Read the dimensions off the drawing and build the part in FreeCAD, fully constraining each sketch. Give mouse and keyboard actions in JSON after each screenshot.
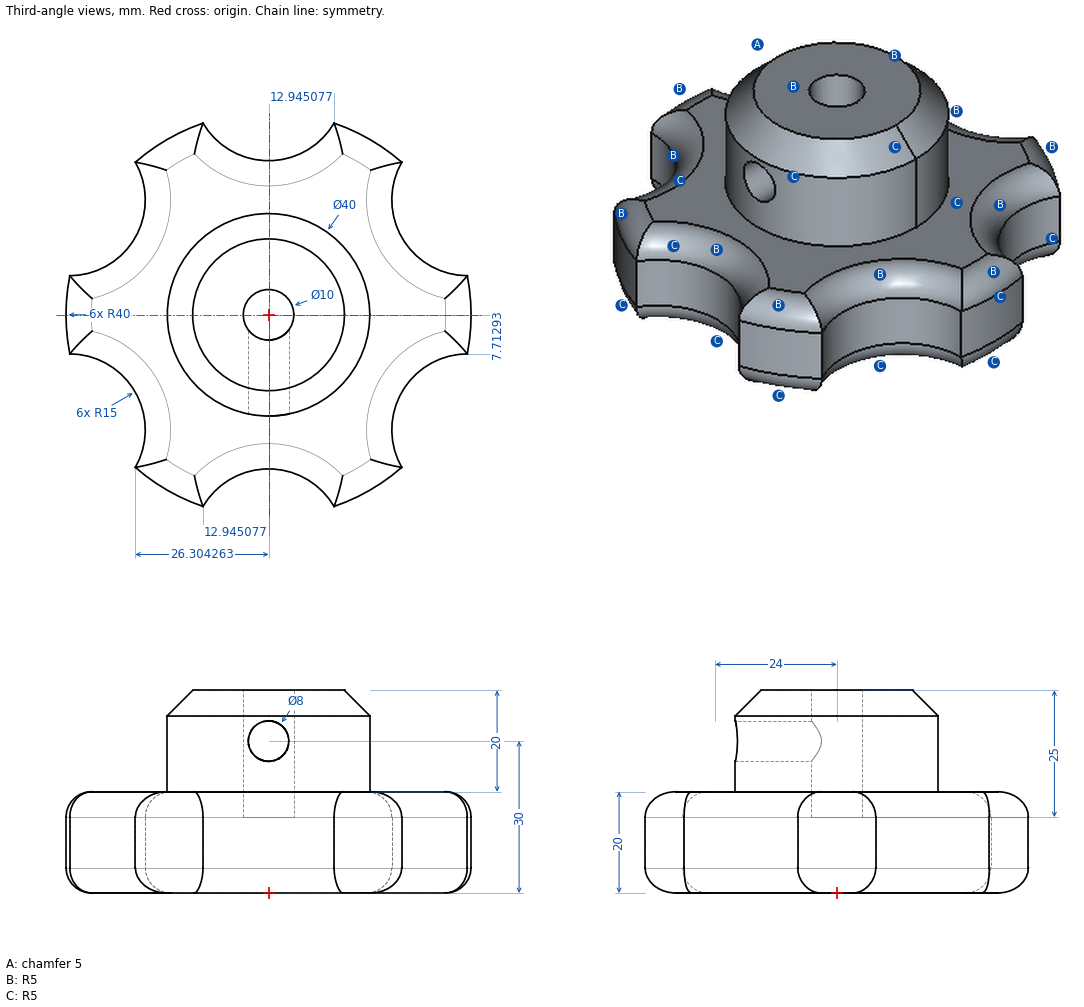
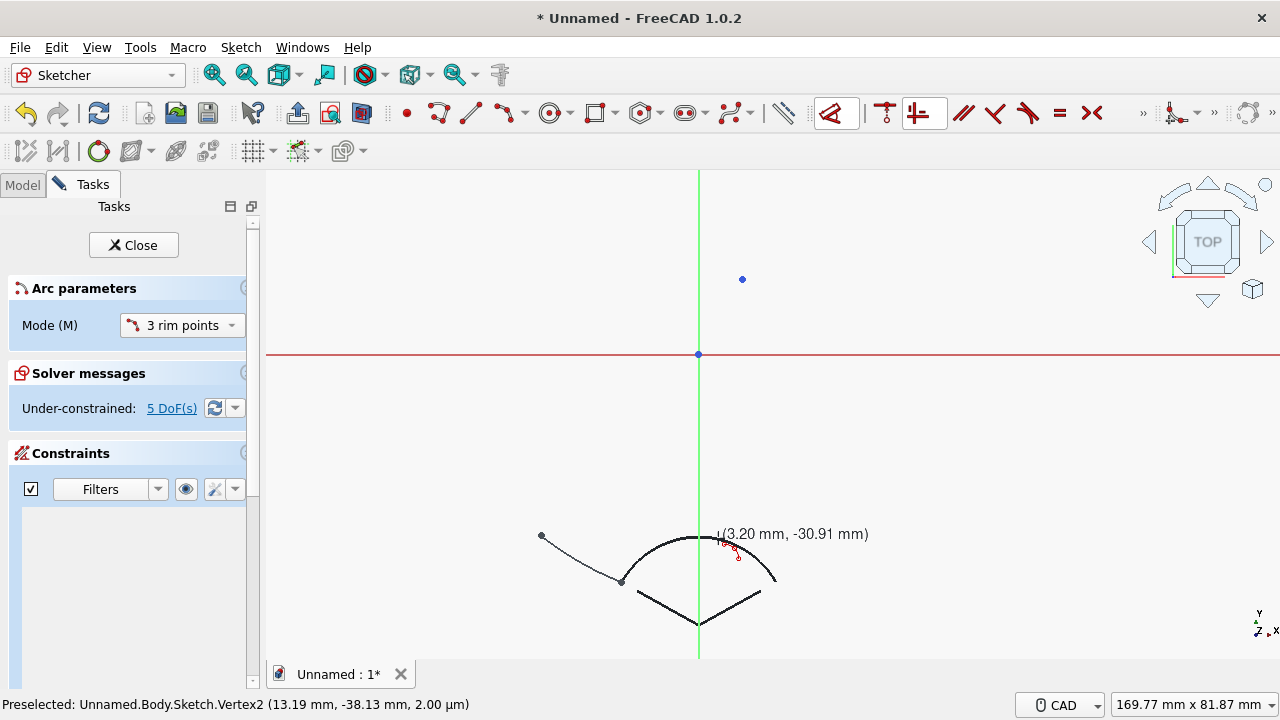
{"action": "left_click", "coordinate": [717, 538]}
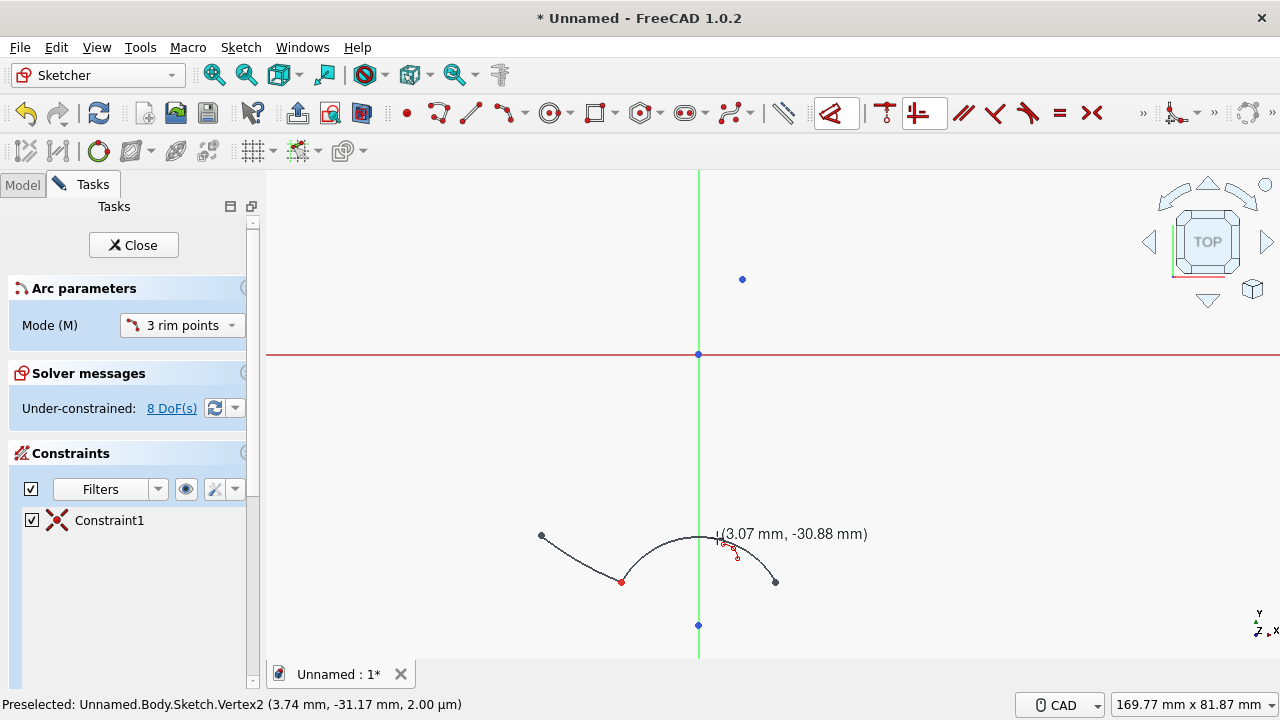
{"action": "left_click", "coordinate": [776, 582]}
{"action": "left_click", "coordinate": [856, 535]}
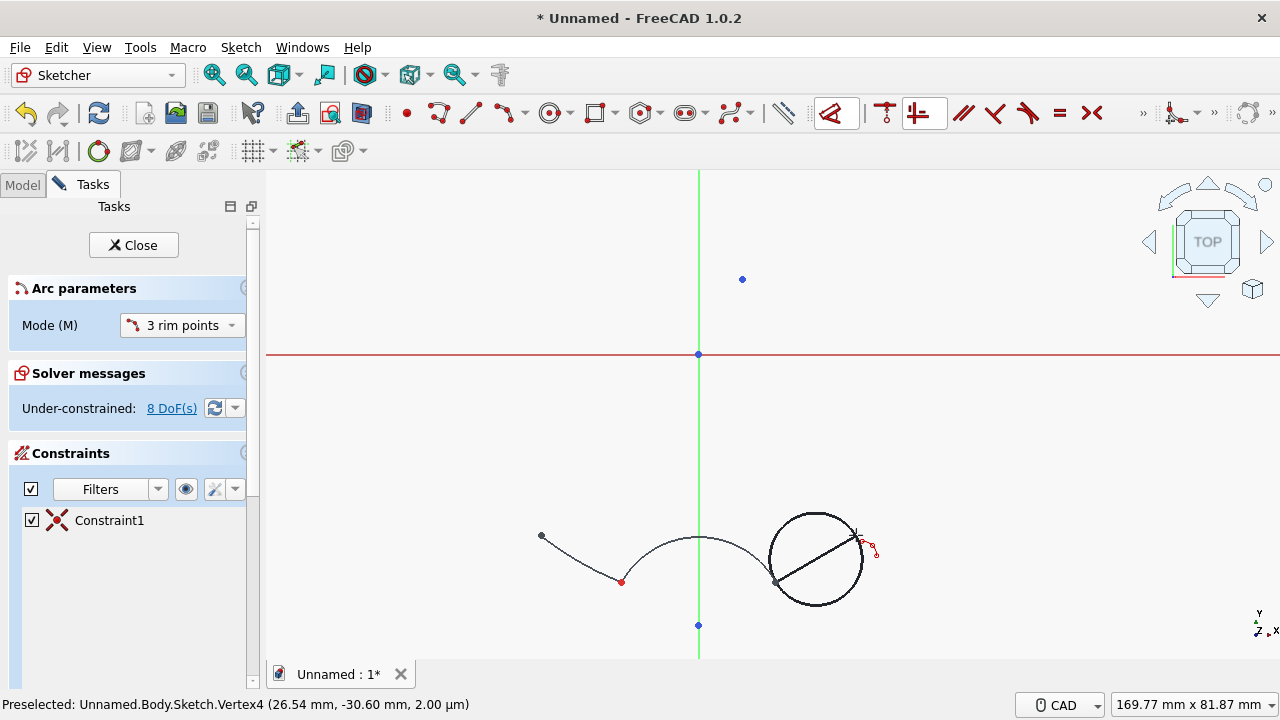
{"action": "scroll", "coordinate": [818, 561], "scroll_direction": "up", "scroll_amount": 7}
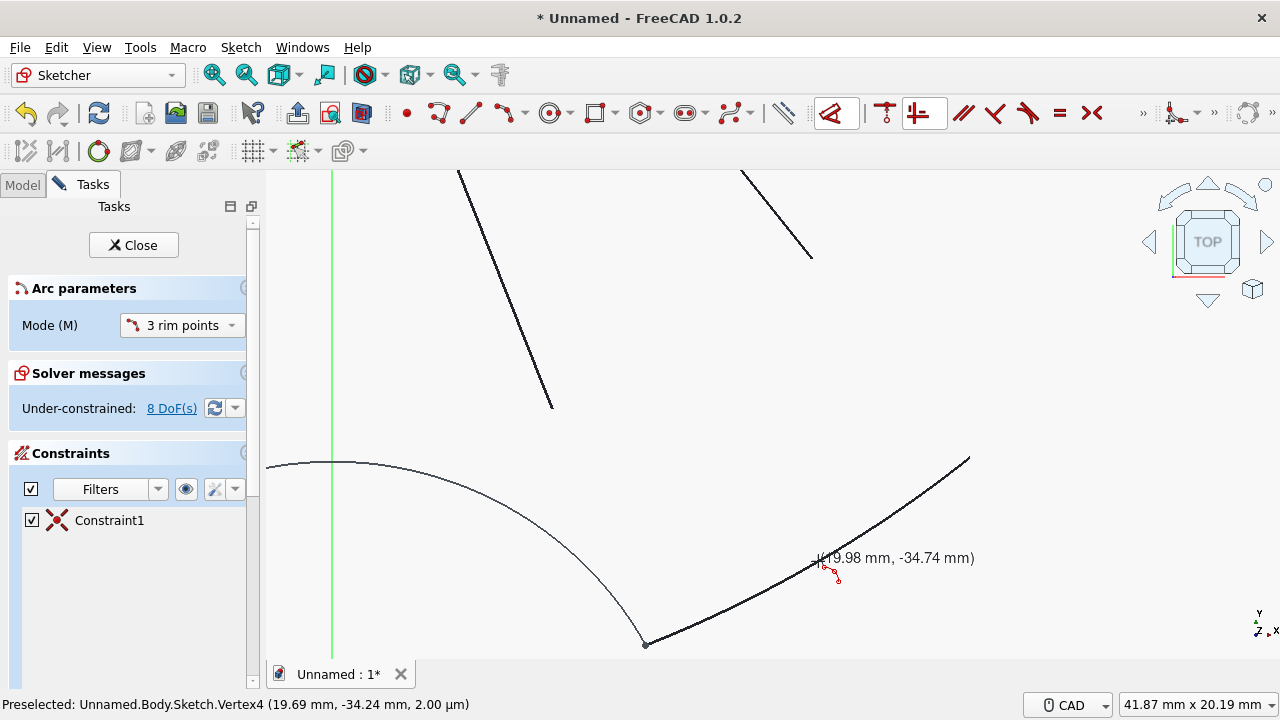
{"action": "left_click", "coordinate": [817, 560]}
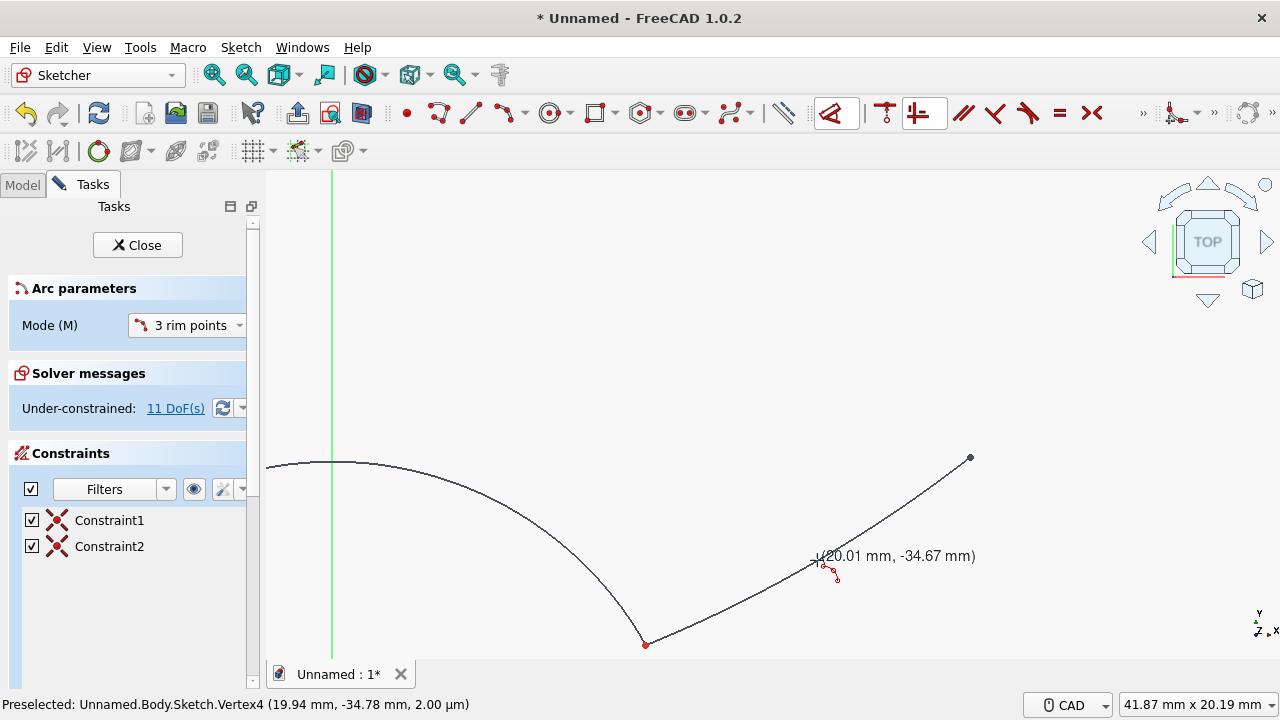
{"action": "scroll", "coordinate": [778, 552], "scroll_direction": "down", "scroll_amount": 9}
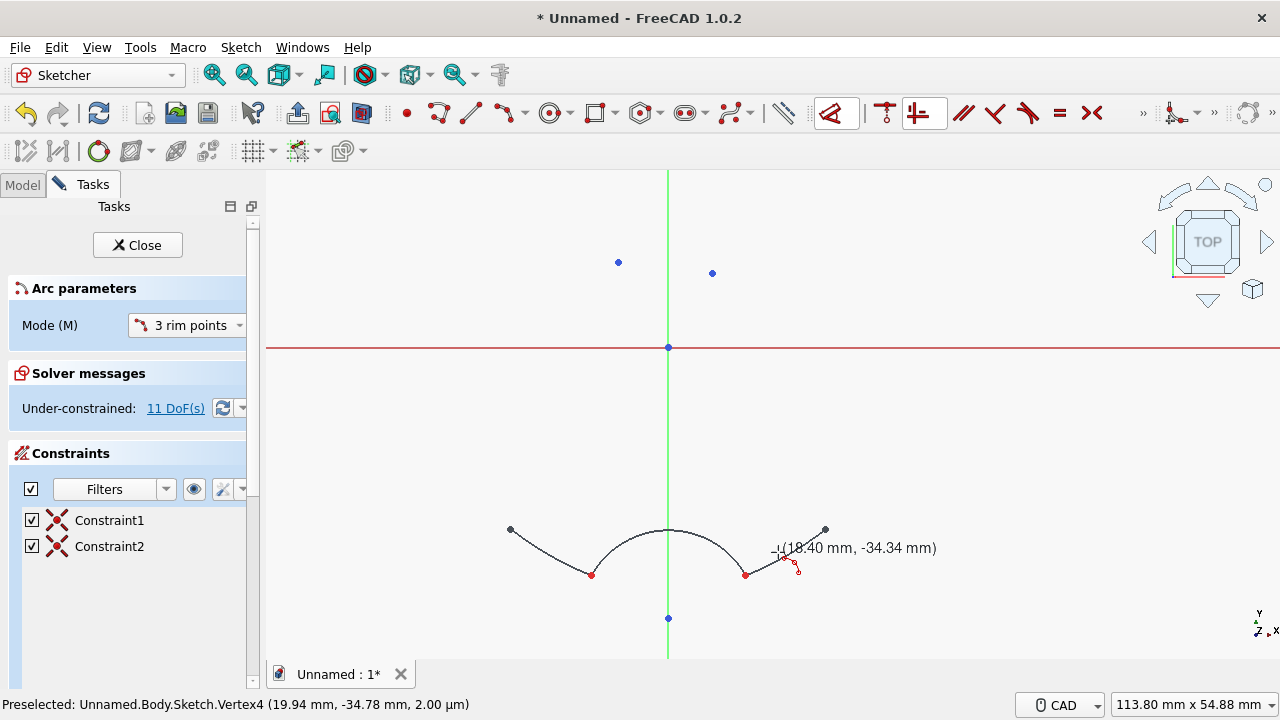
{"action": "left_click", "coordinate": [810, 537]}
{"action": "left_click", "coordinate": [862, 446]}
{"action": "left_click", "coordinate": [810, 476]}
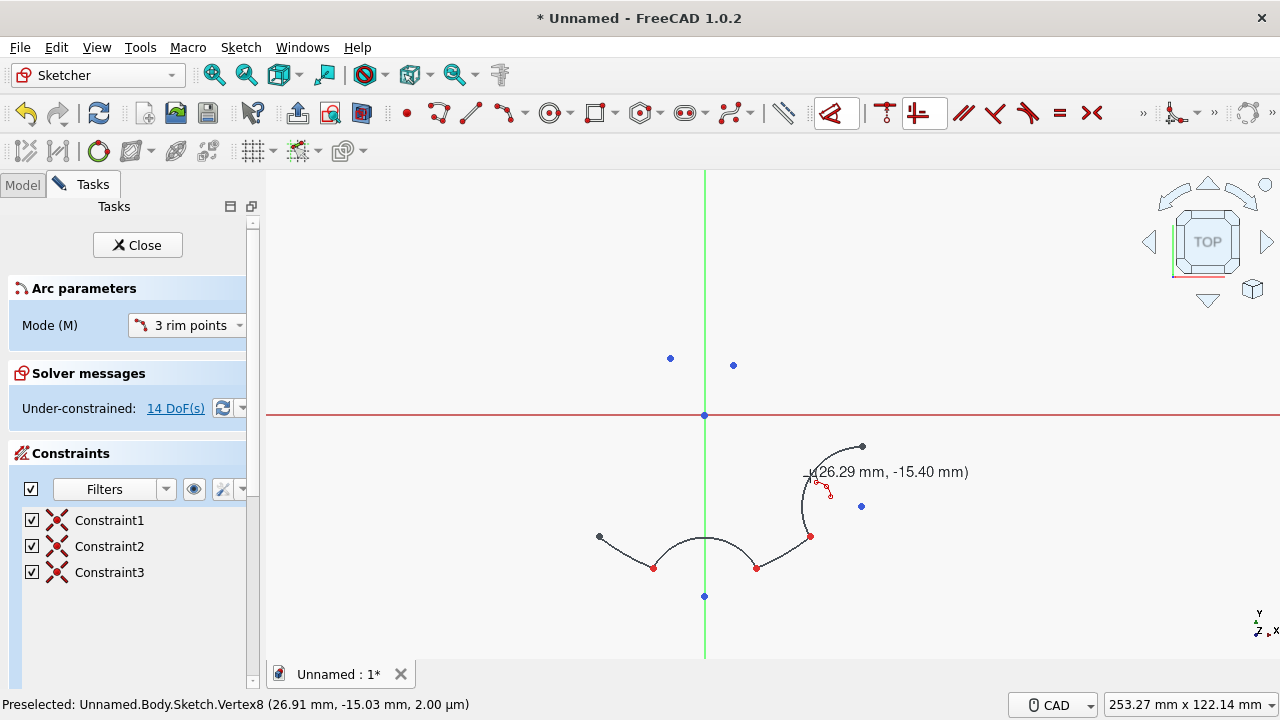
{"action": "left_click", "coordinate": [862, 447]}
{"action": "left_click", "coordinate": [862, 384]}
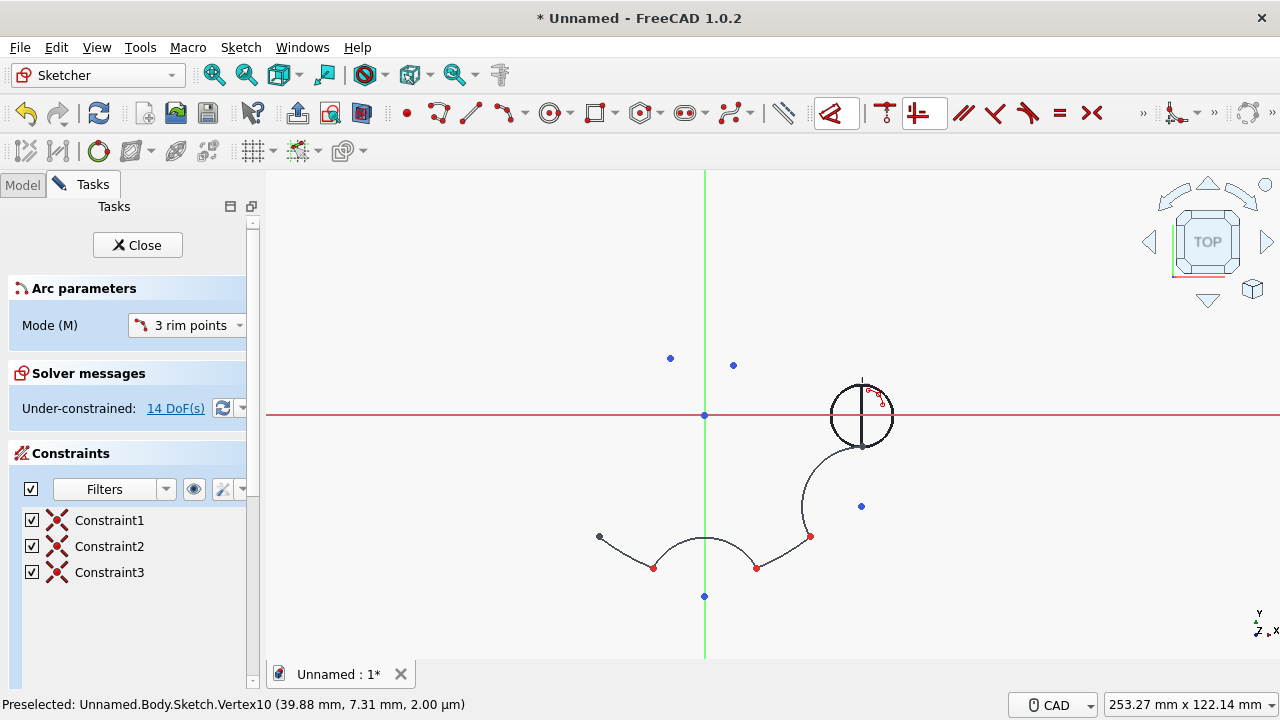
{"action": "scroll", "coordinate": [865, 422], "scroll_direction": "up", "scroll_amount": 9}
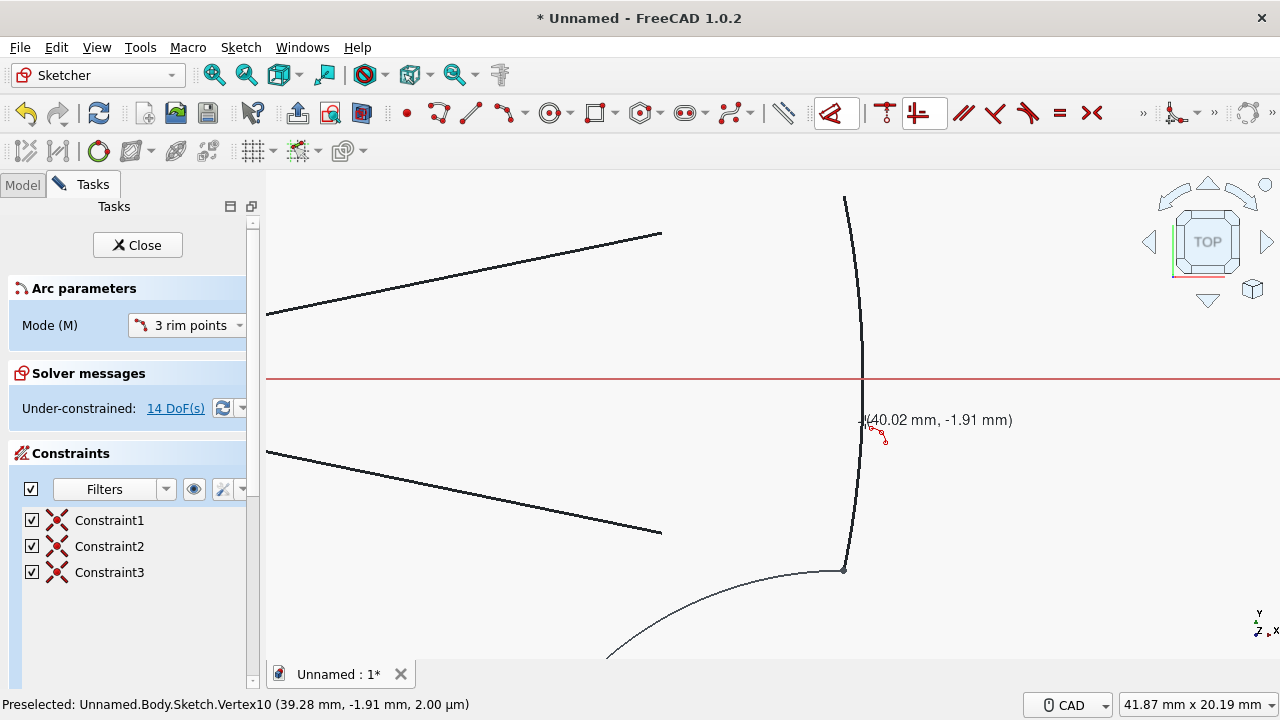
{"action": "left_click", "coordinate": [861, 417]}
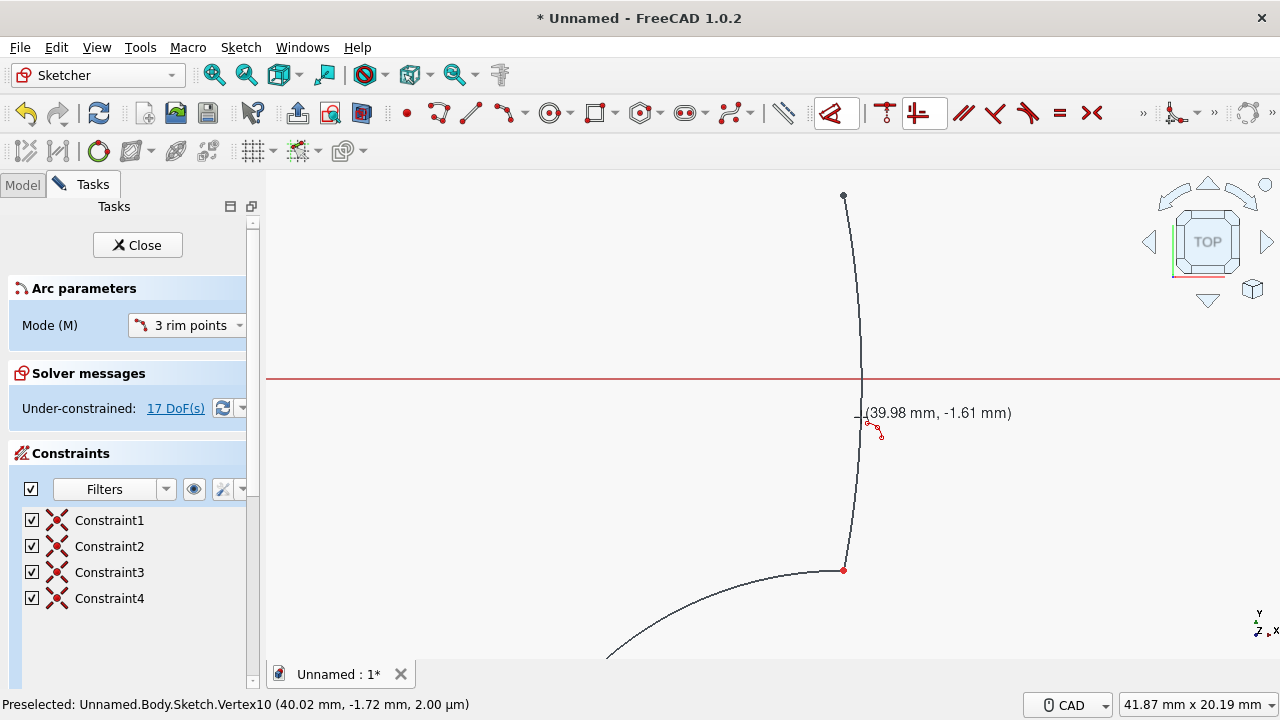
{"action": "scroll", "coordinate": [865, 422], "scroll_direction": "down", "scroll_amount": 9}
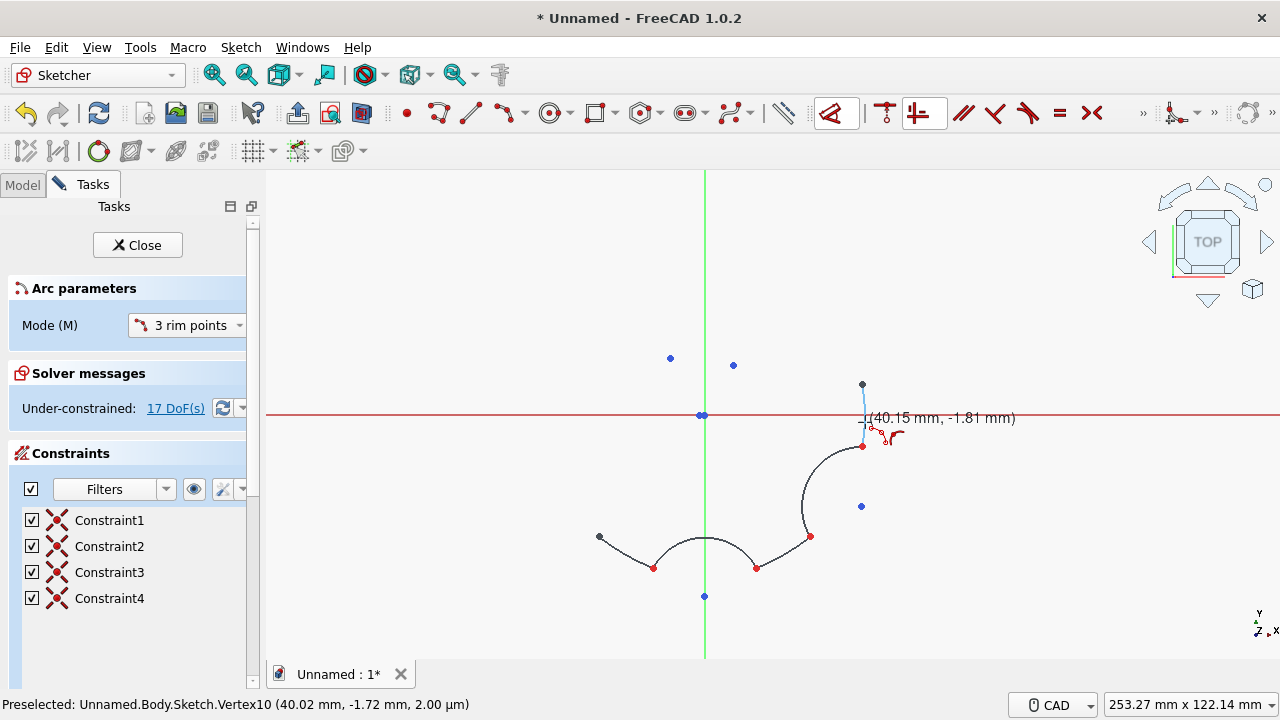
{"action": "left_click", "coordinate": [862, 385]}
{"action": "left_click", "coordinate": [810, 295]}
{"action": "left_click", "coordinate": [810, 354]}